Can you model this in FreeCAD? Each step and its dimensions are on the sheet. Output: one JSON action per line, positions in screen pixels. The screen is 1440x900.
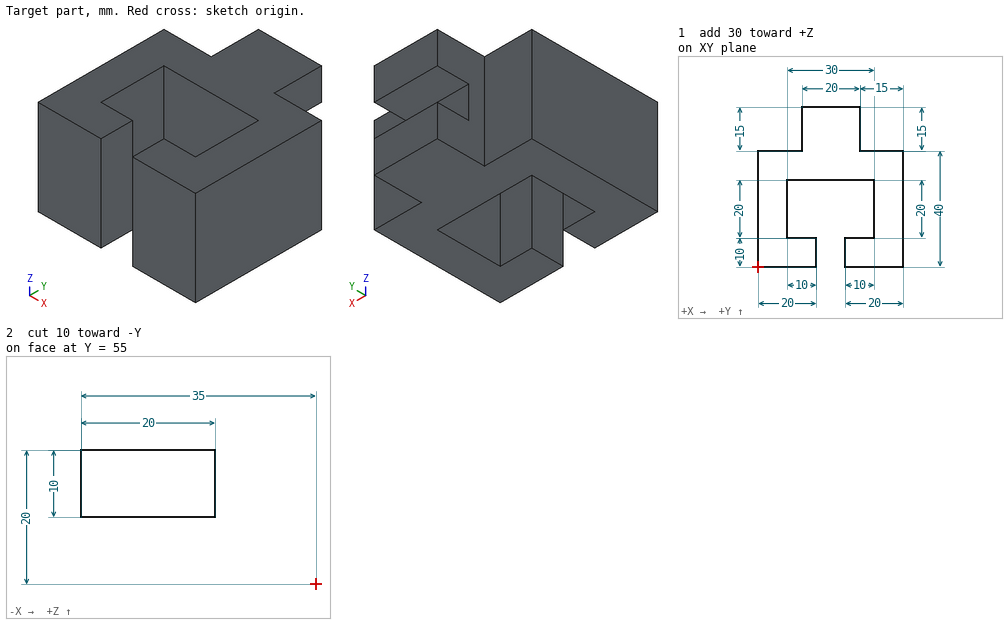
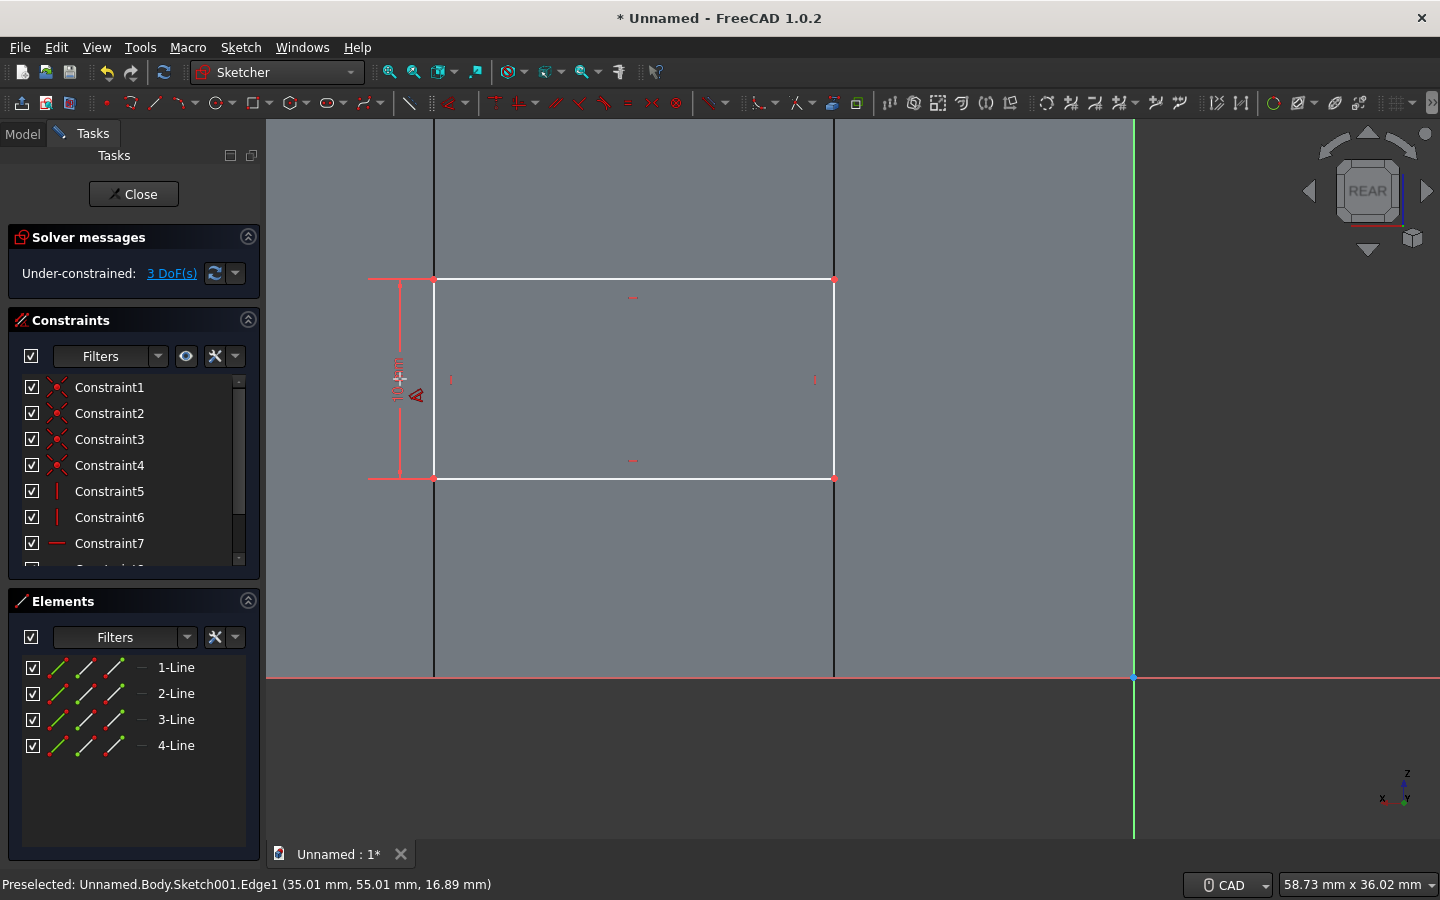
{"action": "left_click", "coordinate": [554, 479]}
{"action": "left_click", "coordinate": [634, 513]}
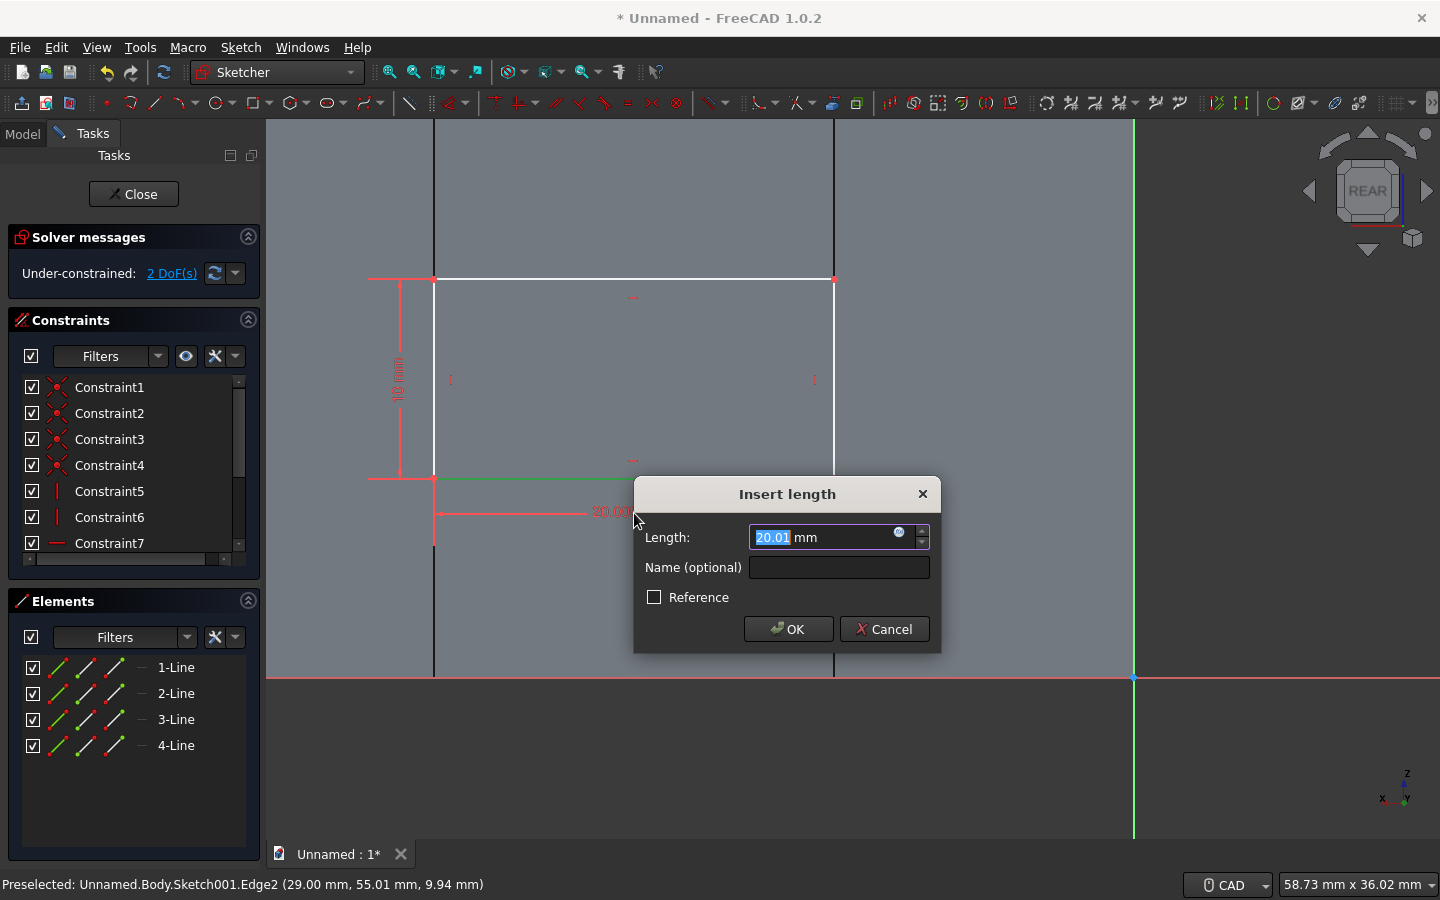
{"action": "type", "text": "20"}
{"action": "key", "text": "Return"}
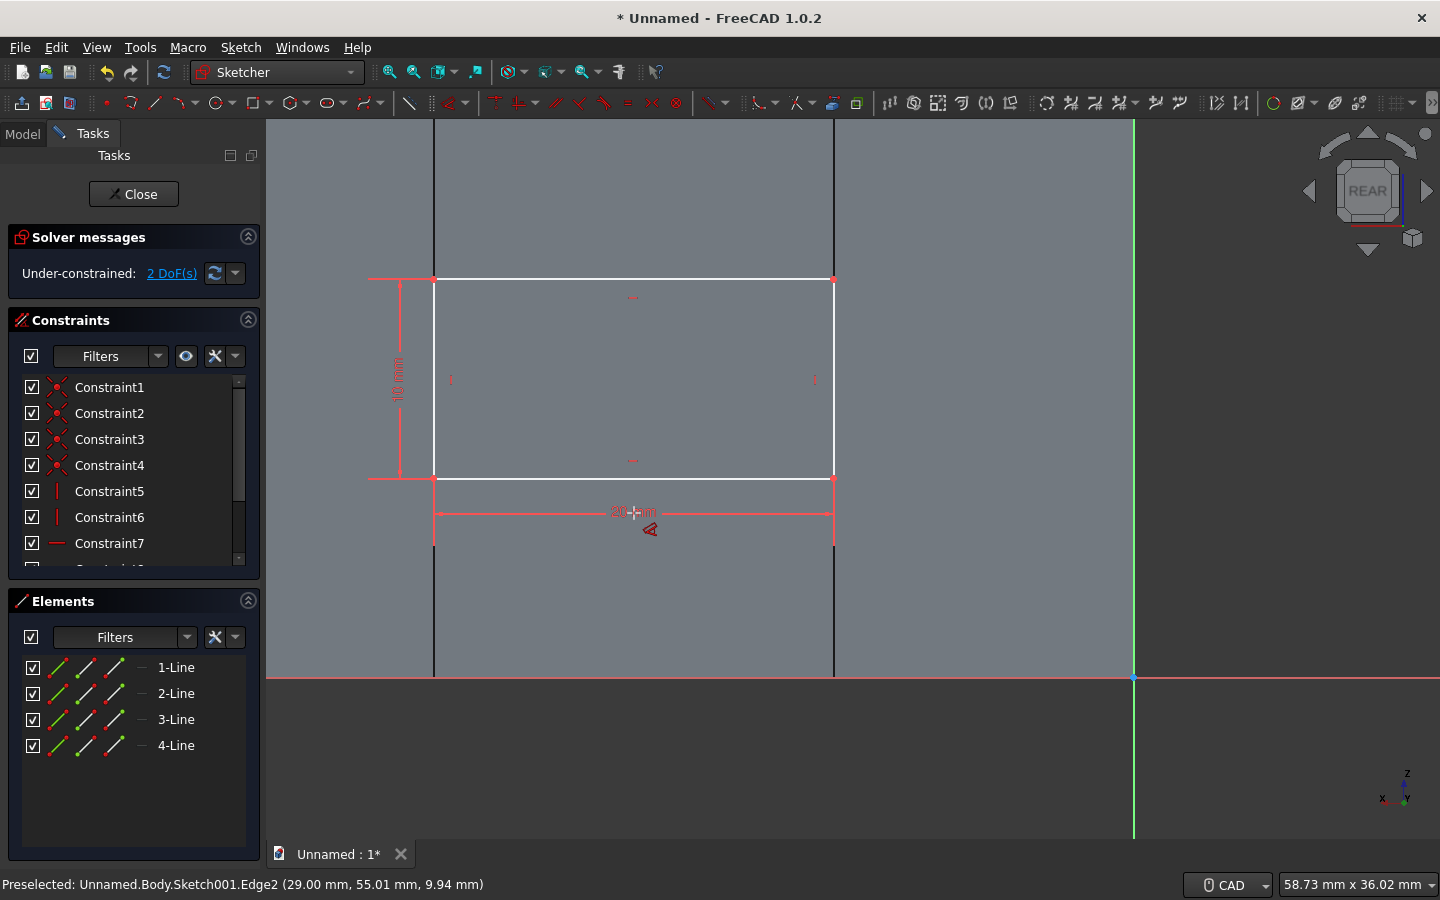
{"action": "left_click", "coordinate": [434, 279]}
{"action": "left_click", "coordinate": [784, 712]}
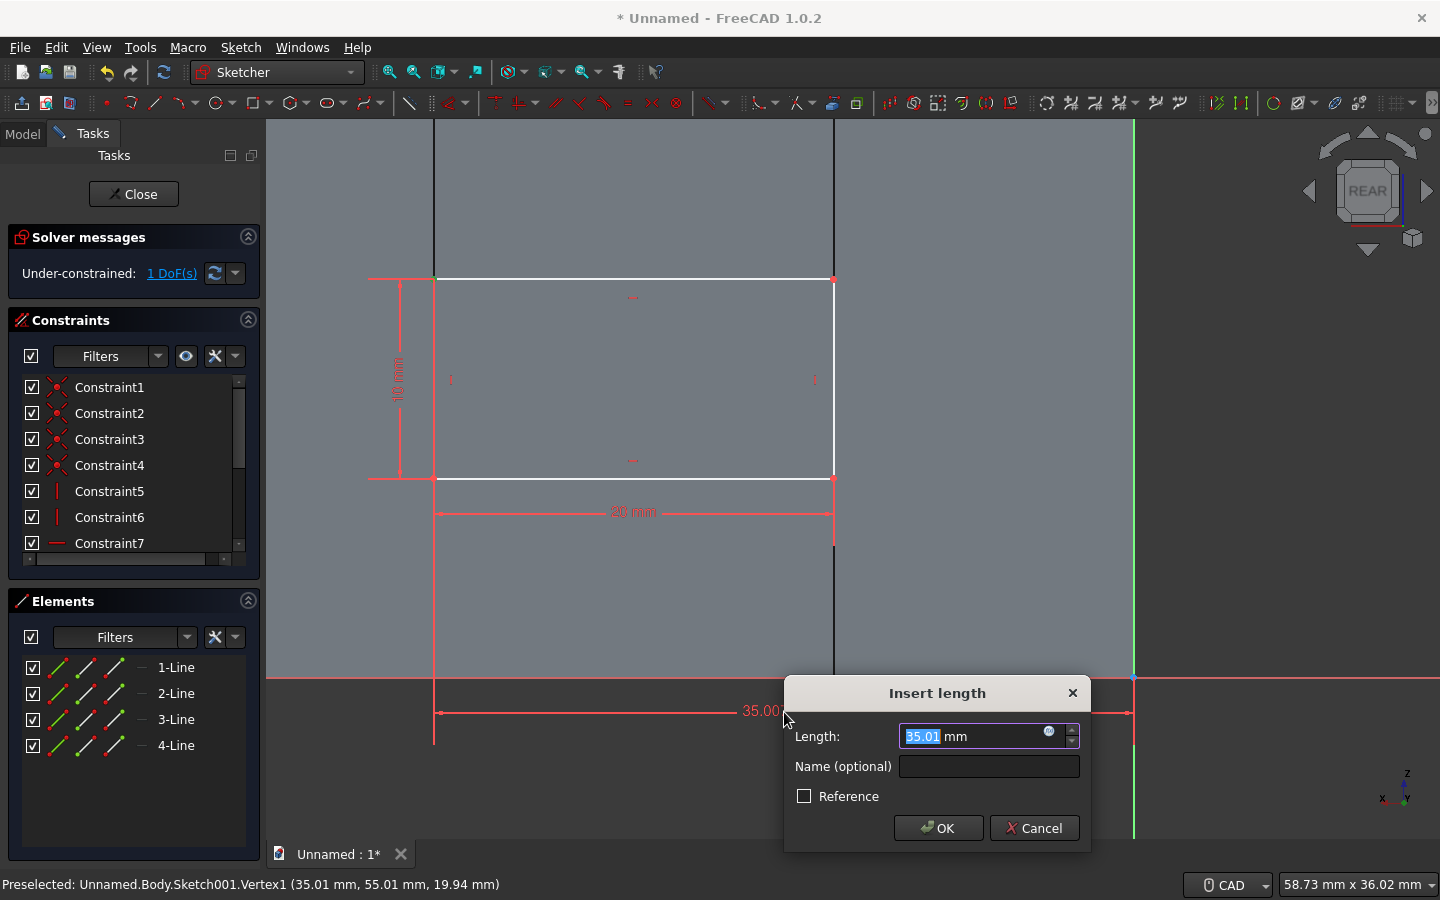
{"action": "type", "text": "35"}
{"action": "key", "text": "Return"}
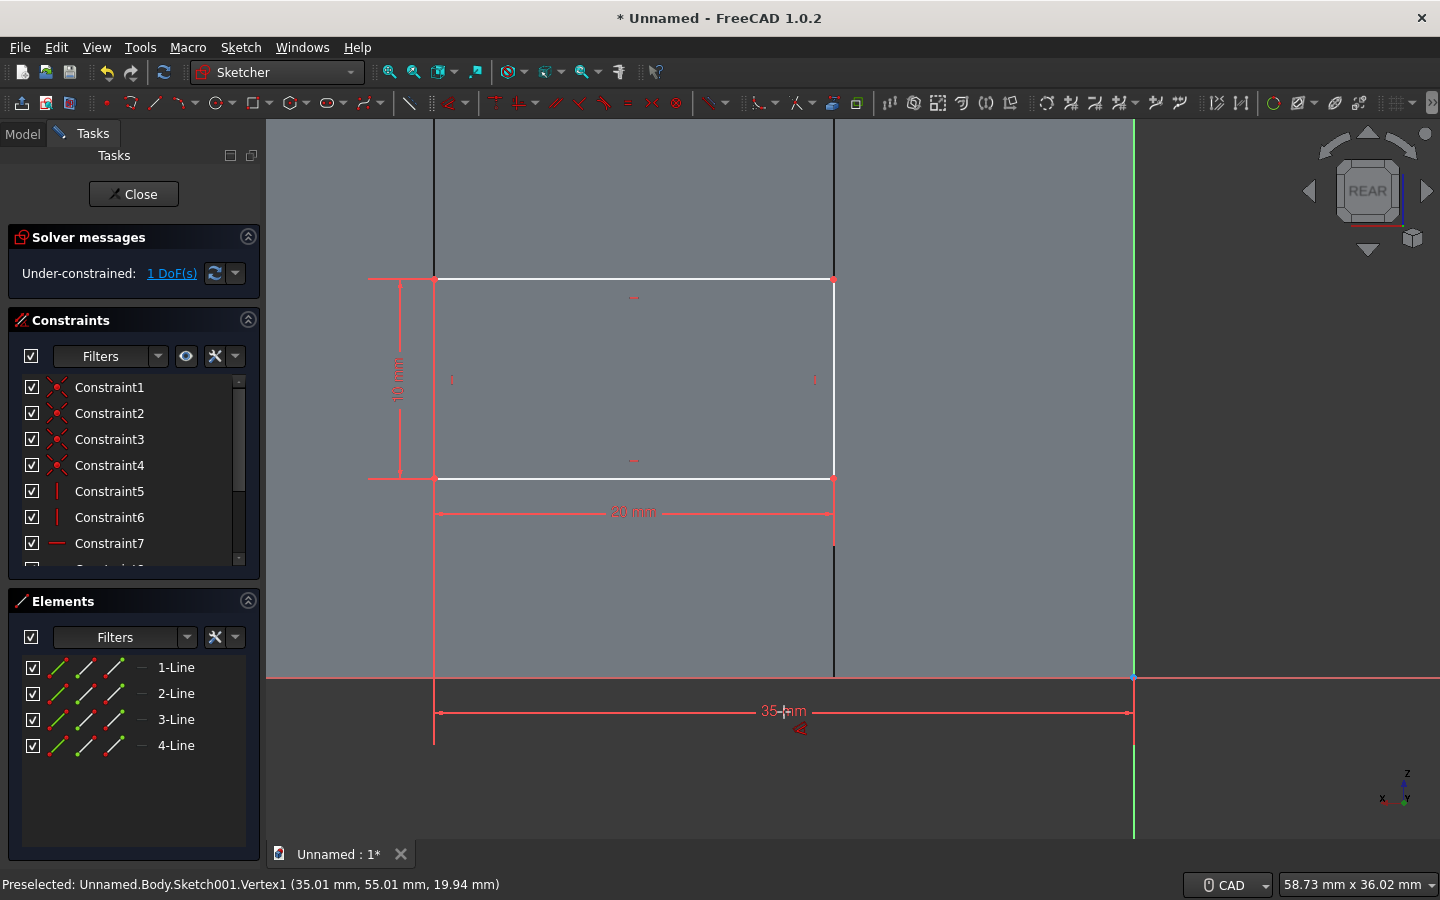
{"action": "left_click", "coordinate": [434, 279]}
{"action": "left_click", "coordinate": [1168, 478]}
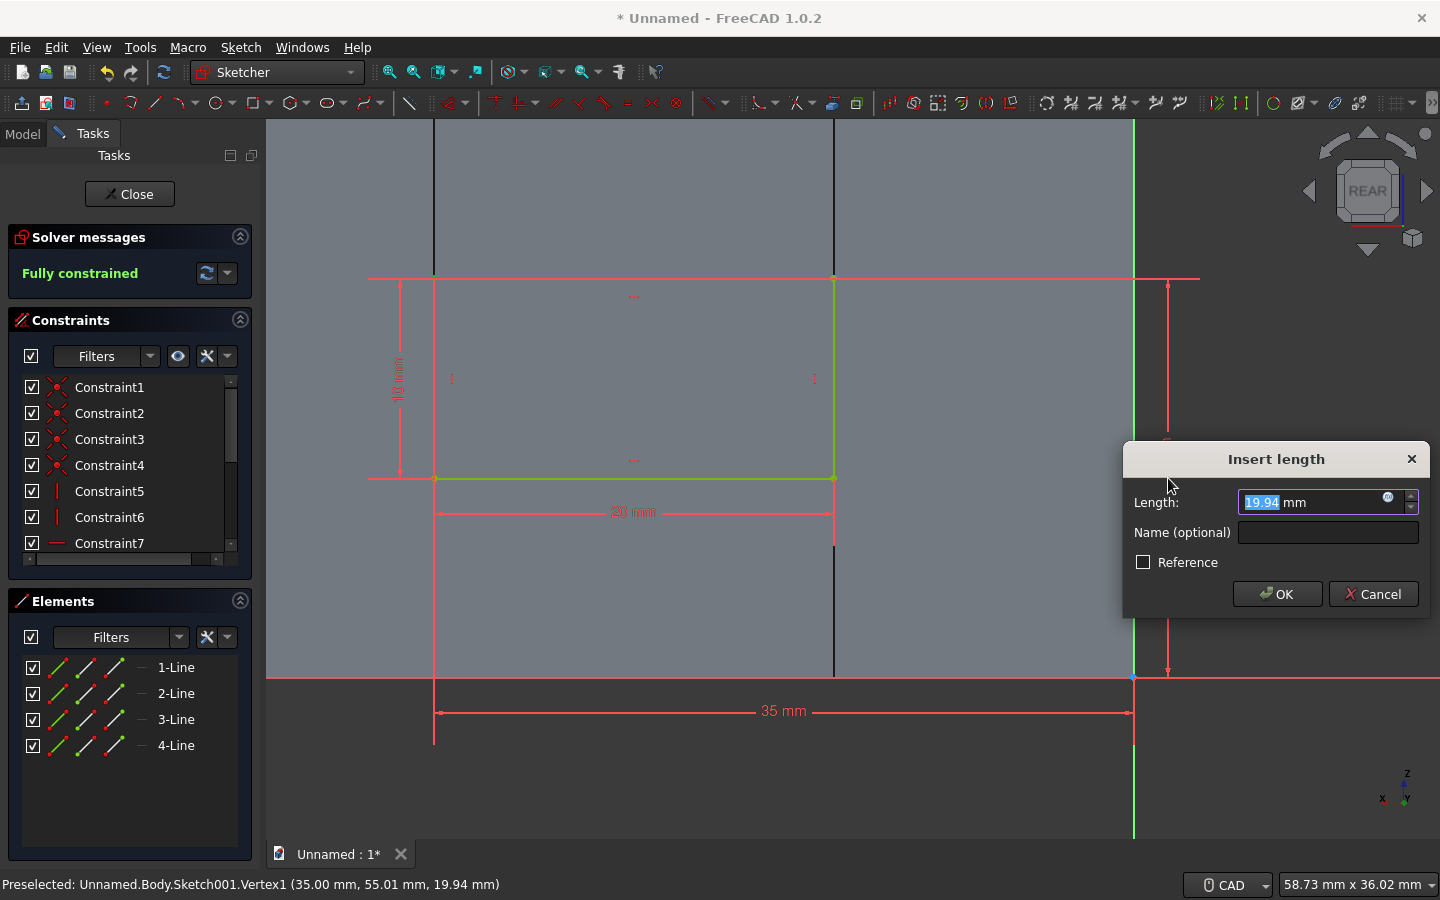
{"action": "type", "text": "20"}
{"action": "key", "text": "Return"}
{"action": "key", "text": "Escape"}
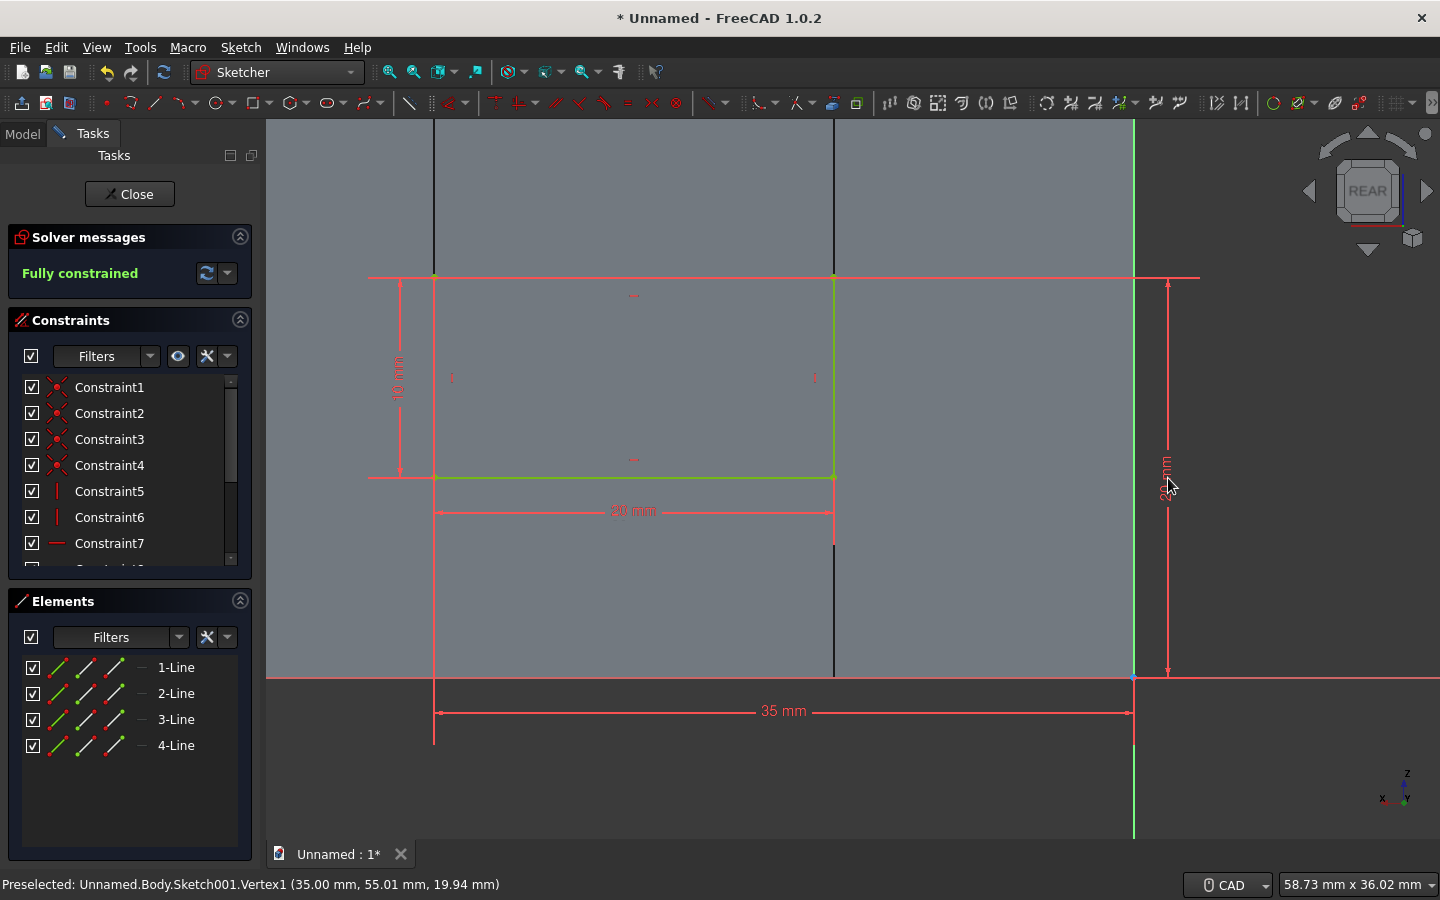
{"action": "left_click", "coordinate": [130, 194]}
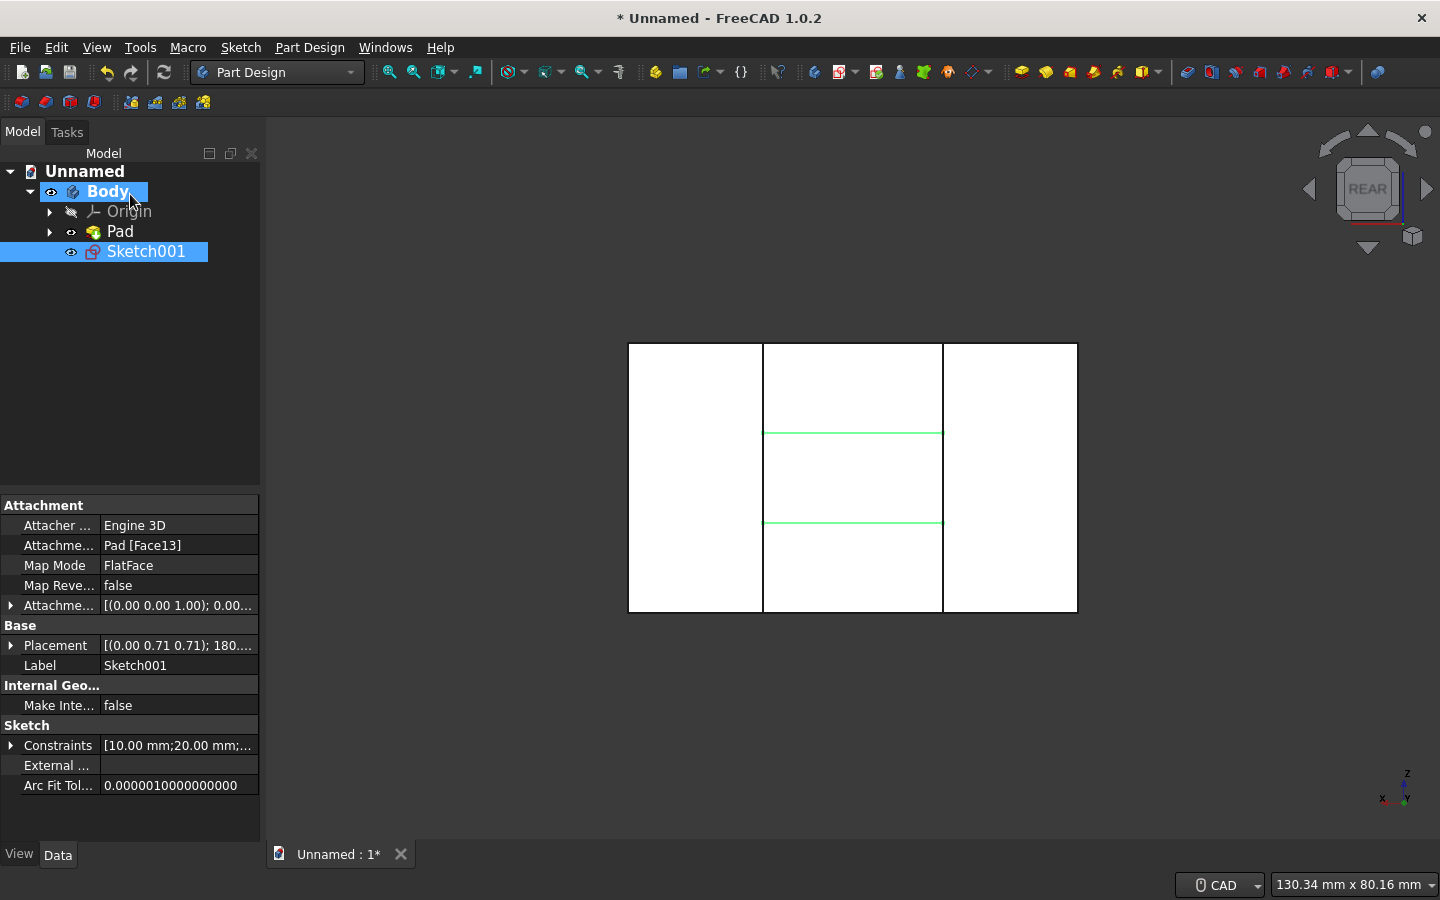
{"action": "left_click", "coordinate": [1188, 72]}